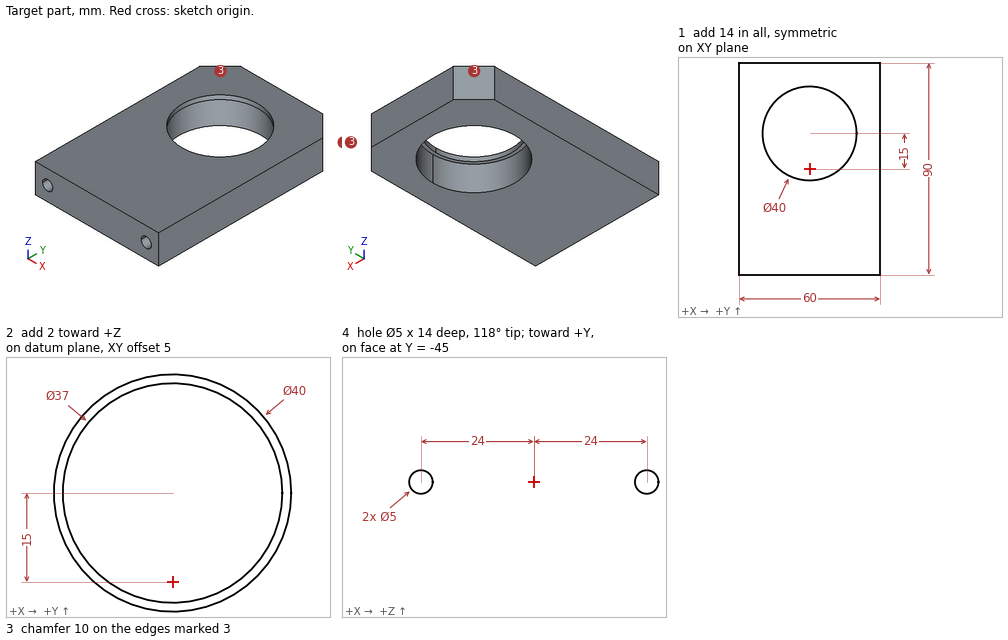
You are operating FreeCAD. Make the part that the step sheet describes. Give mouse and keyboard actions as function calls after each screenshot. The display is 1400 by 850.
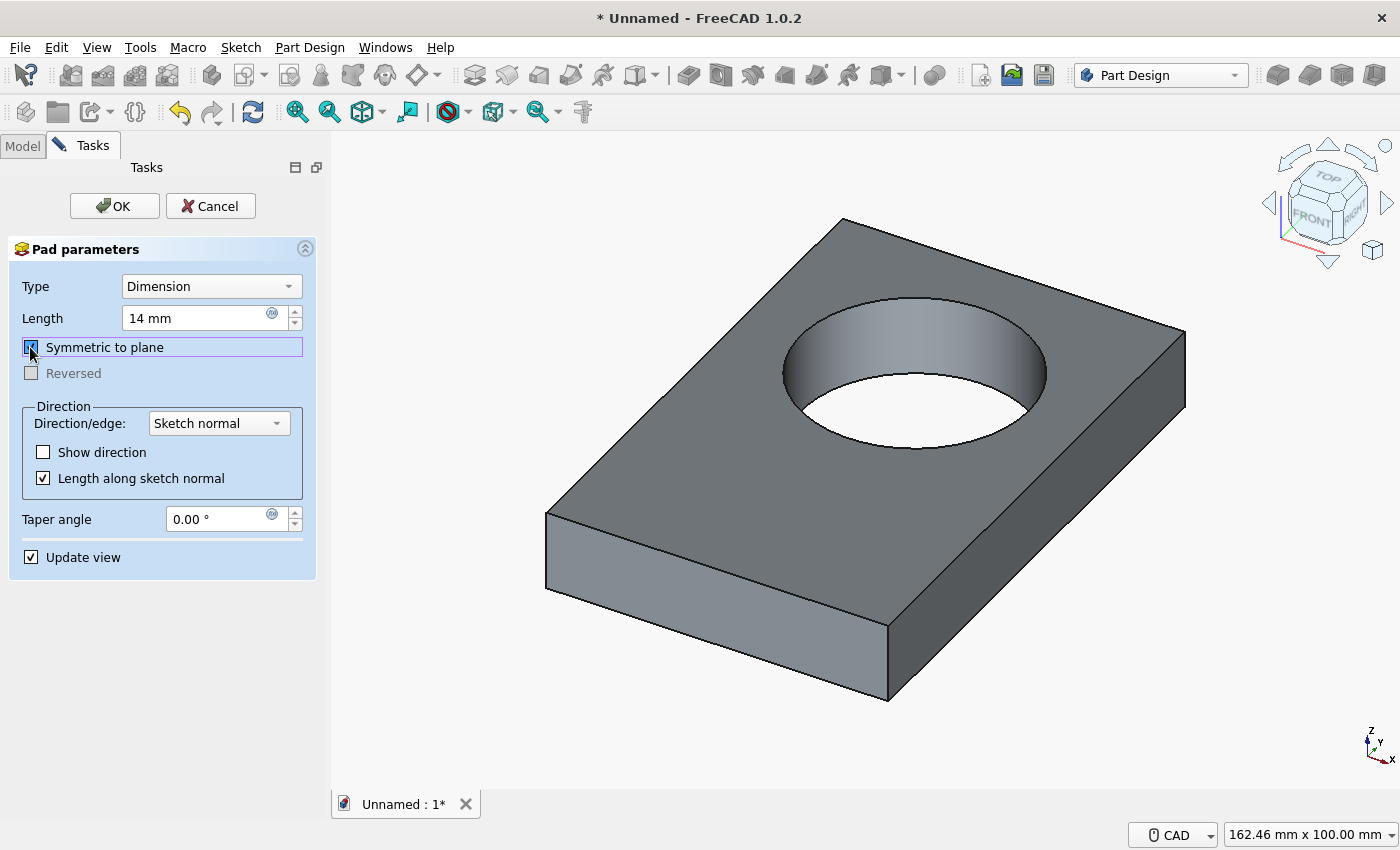
click(115, 206)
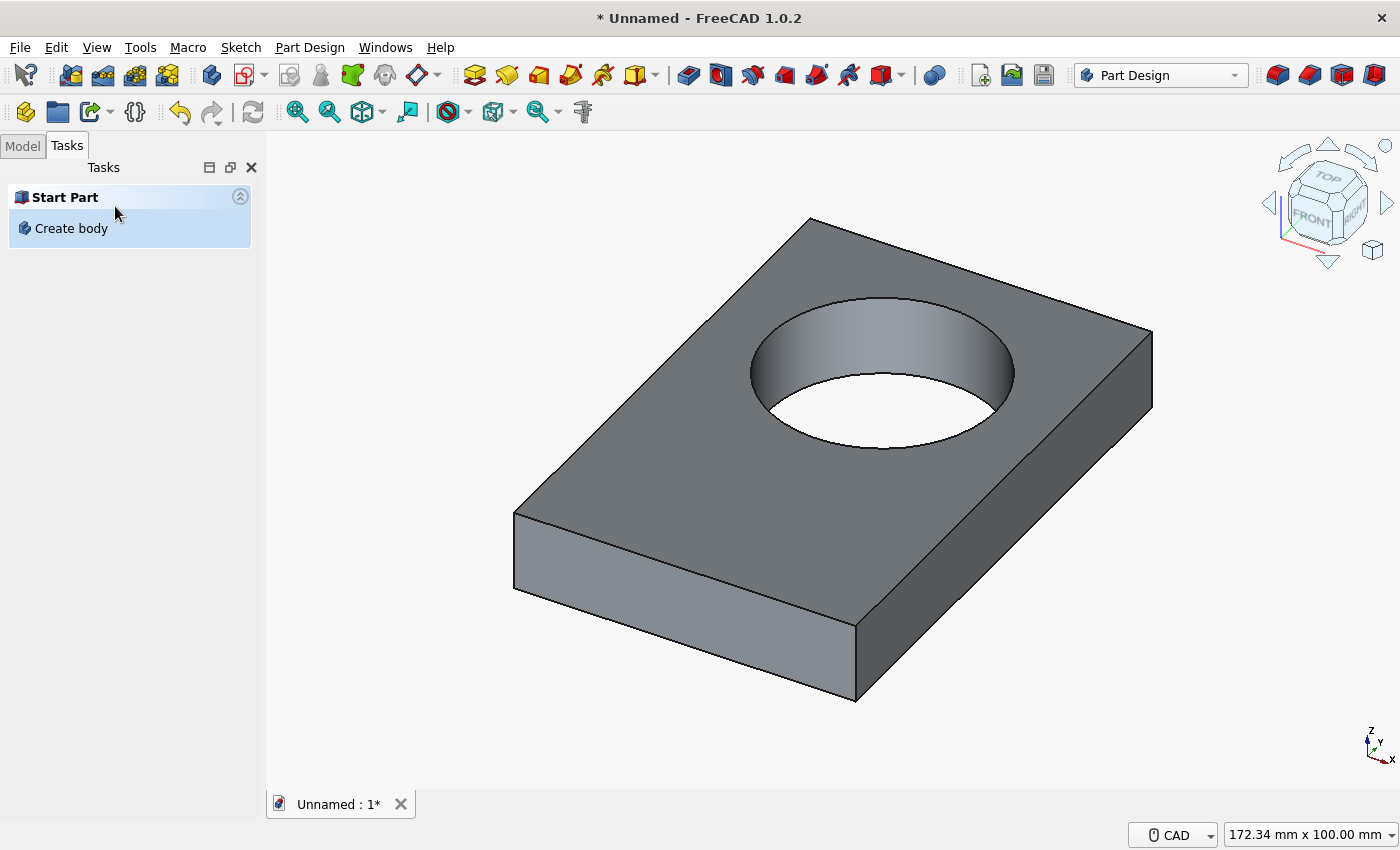
click(23, 145)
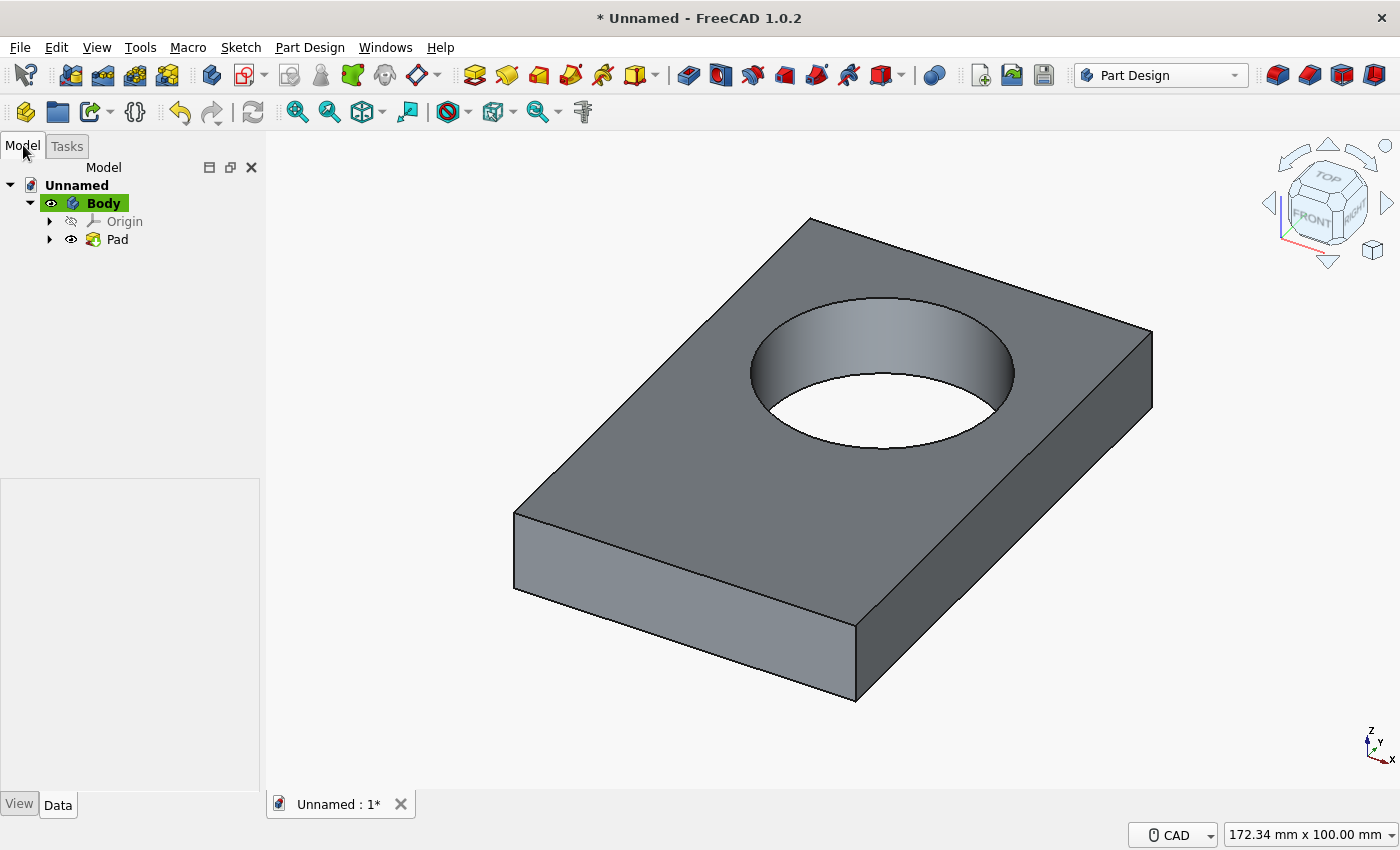
click(50, 221)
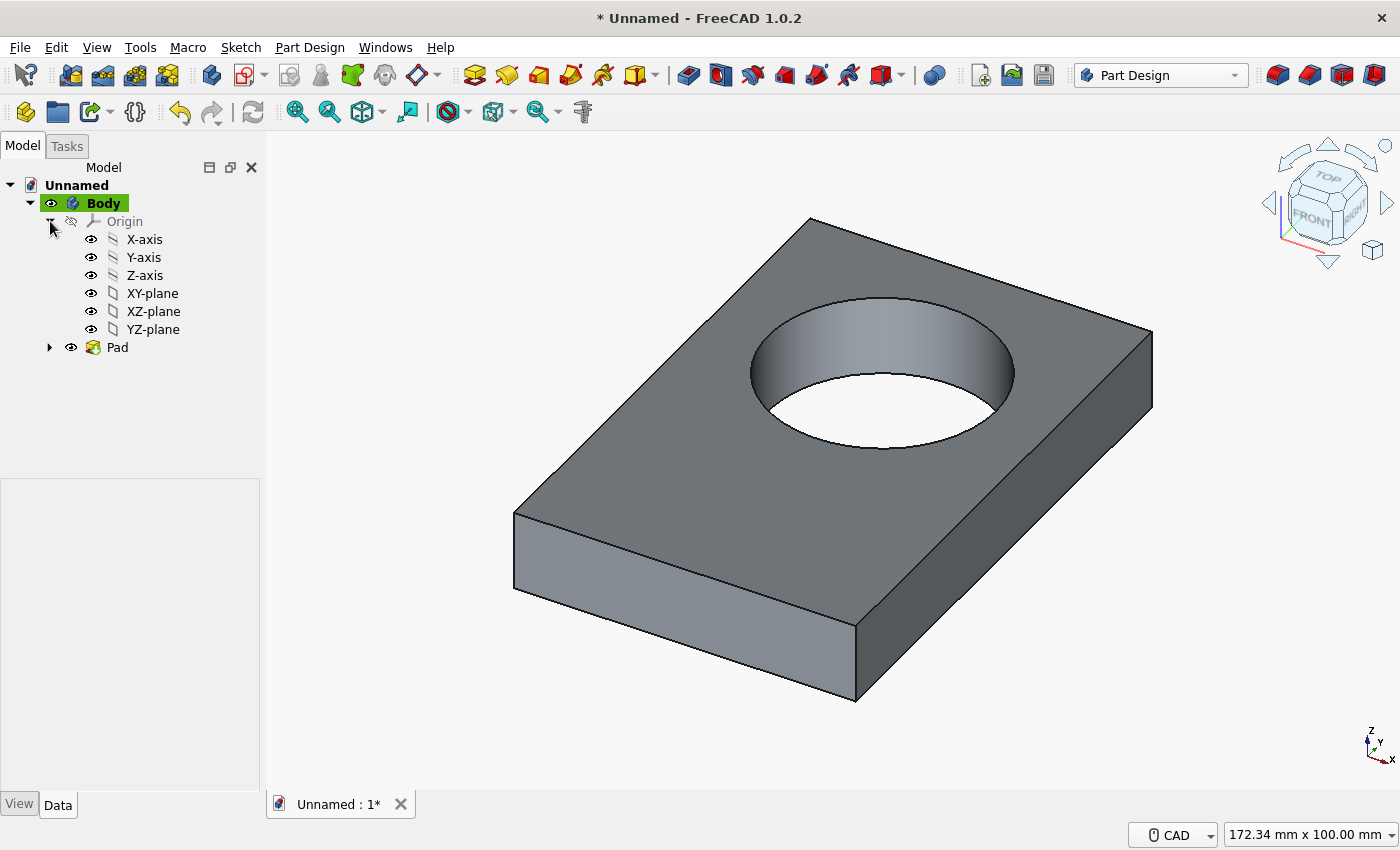
click(136, 293)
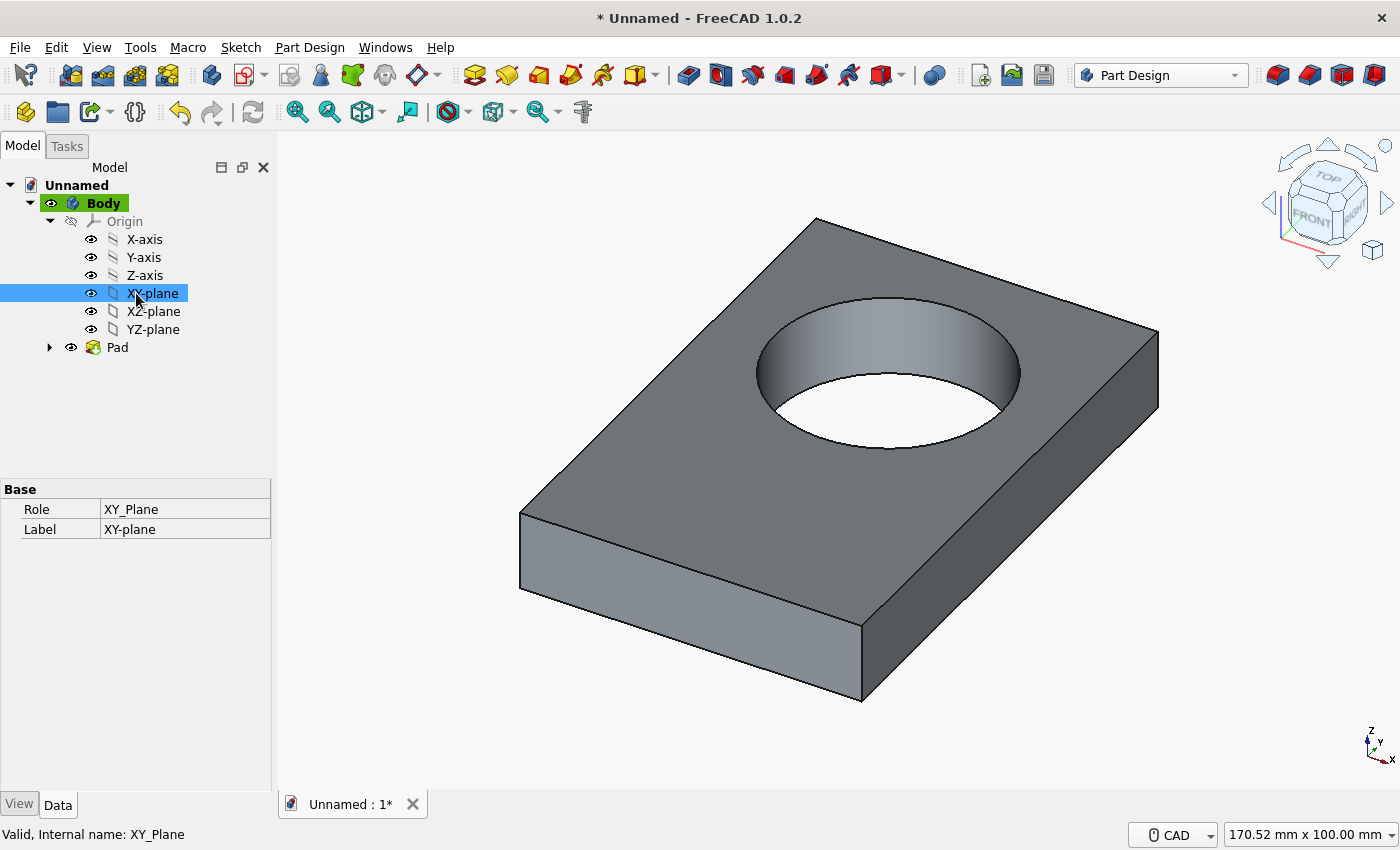
click(418, 76)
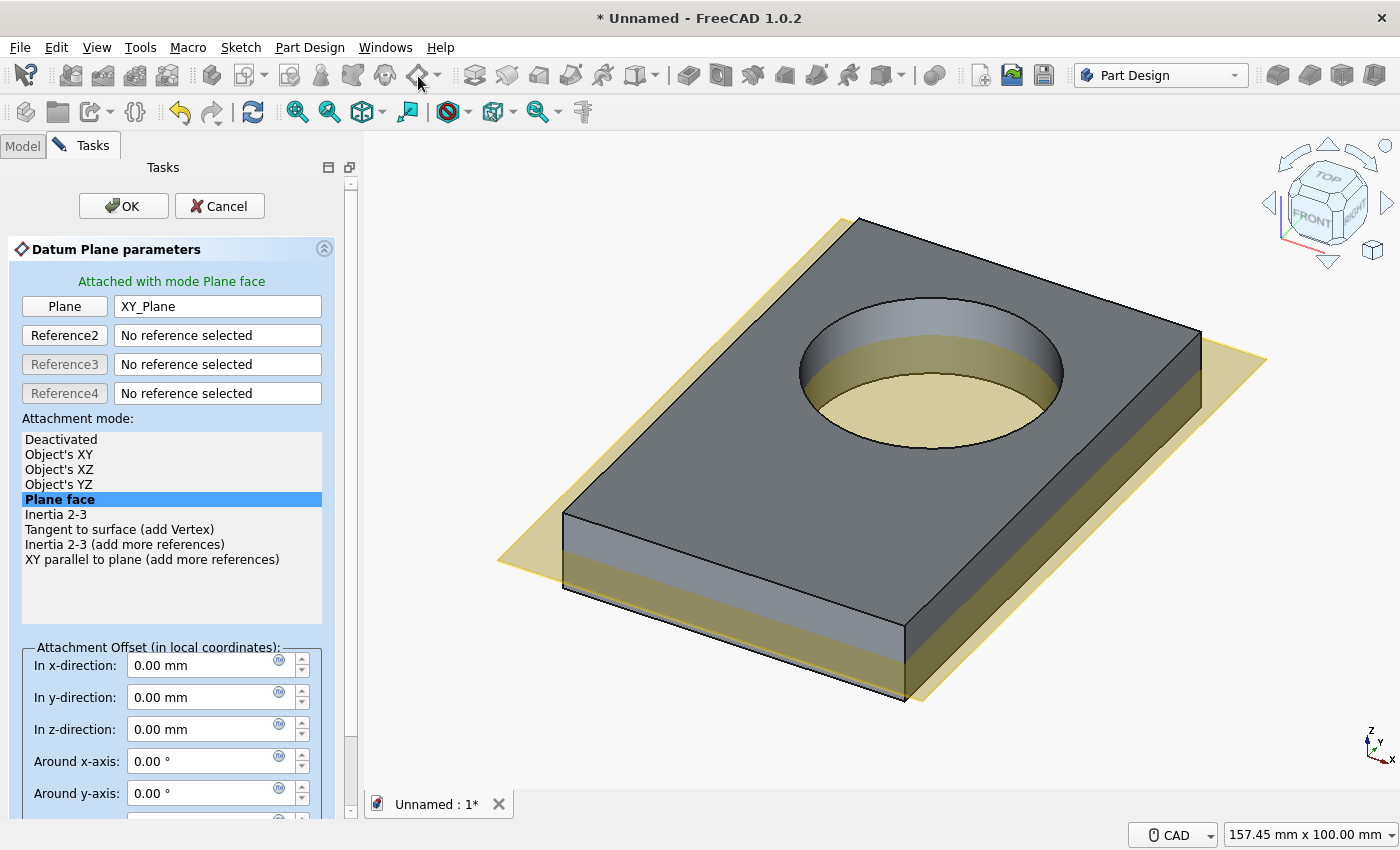
triple_click(210, 729)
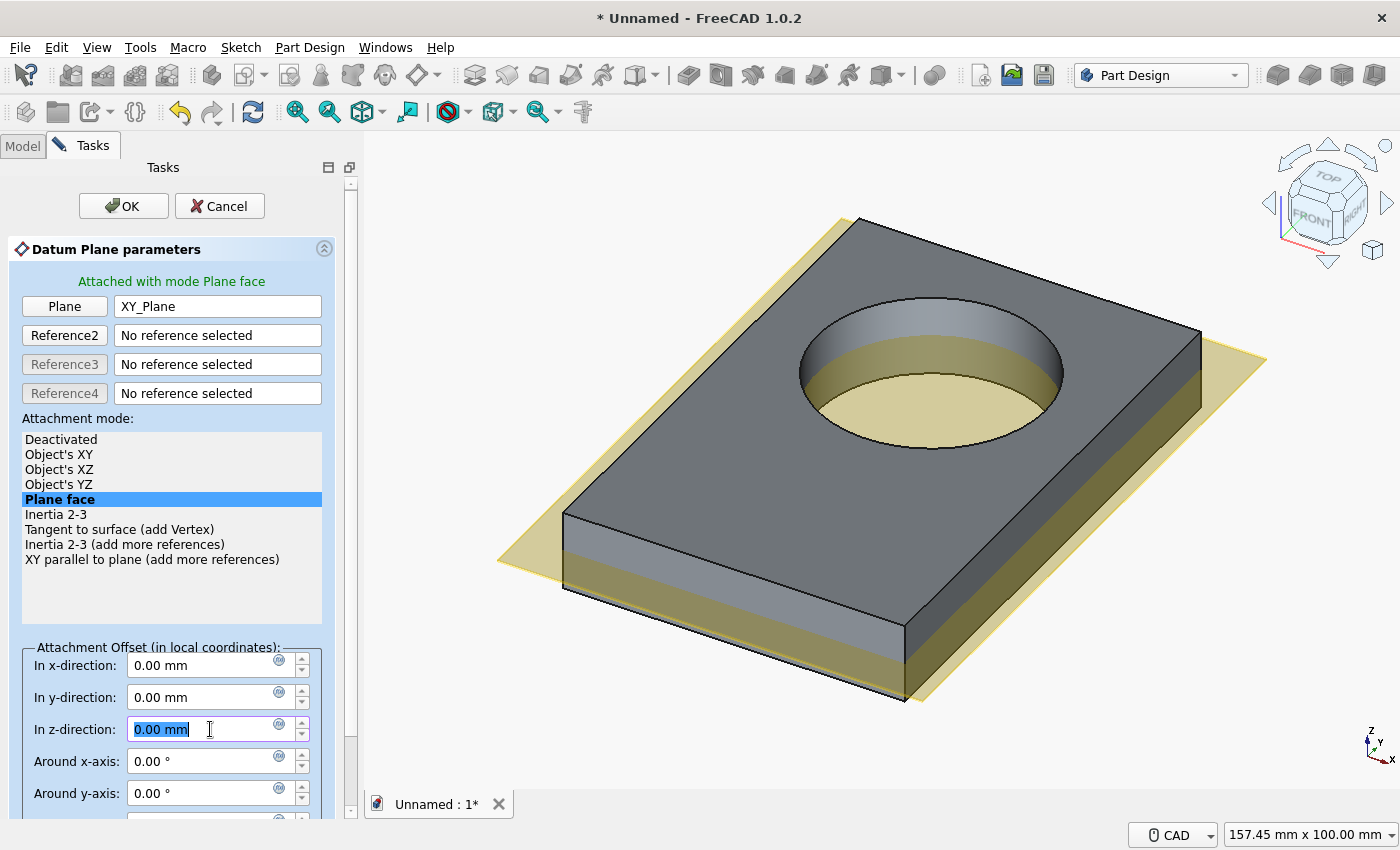
text(5)
key(Tab)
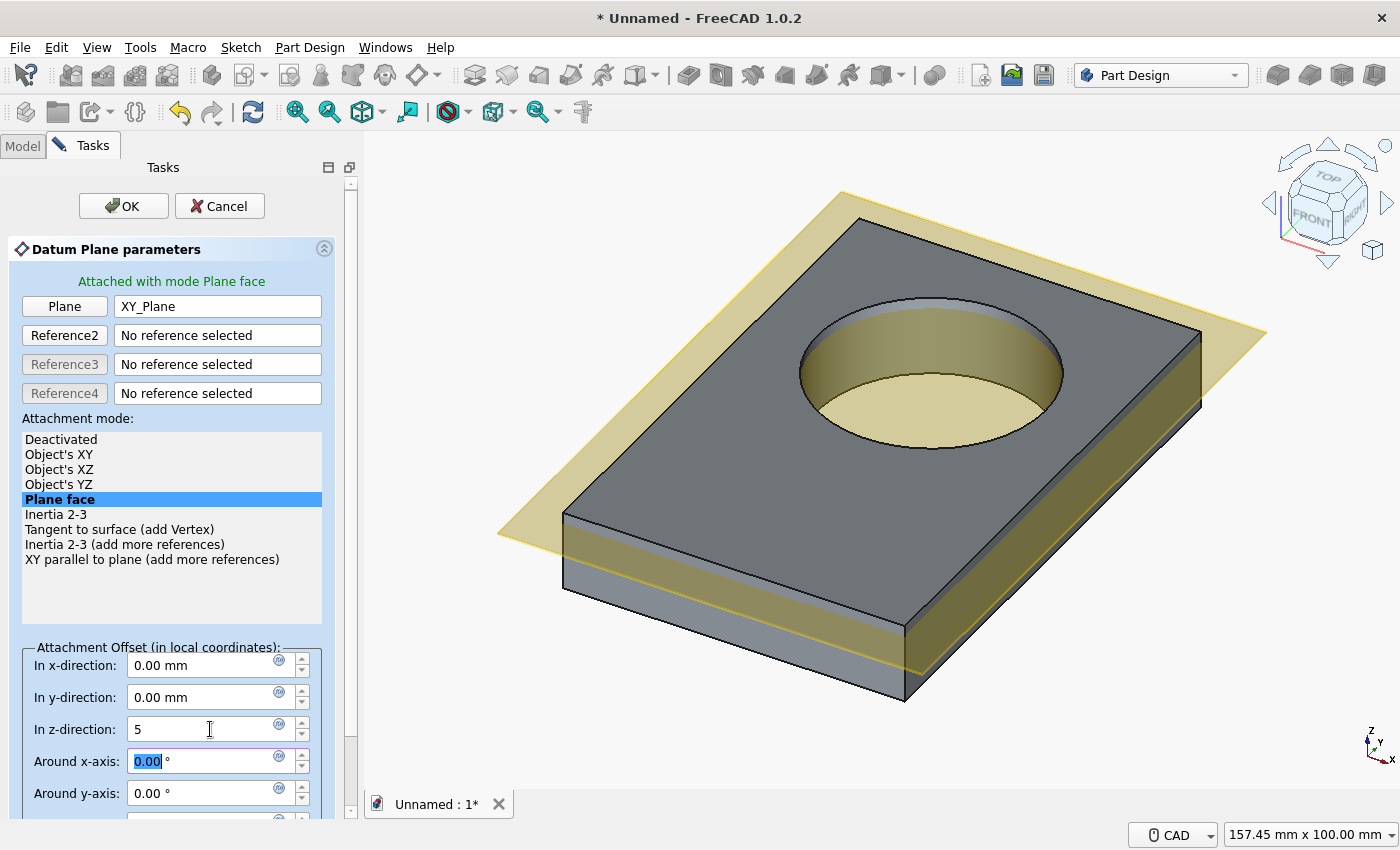
click(124, 206)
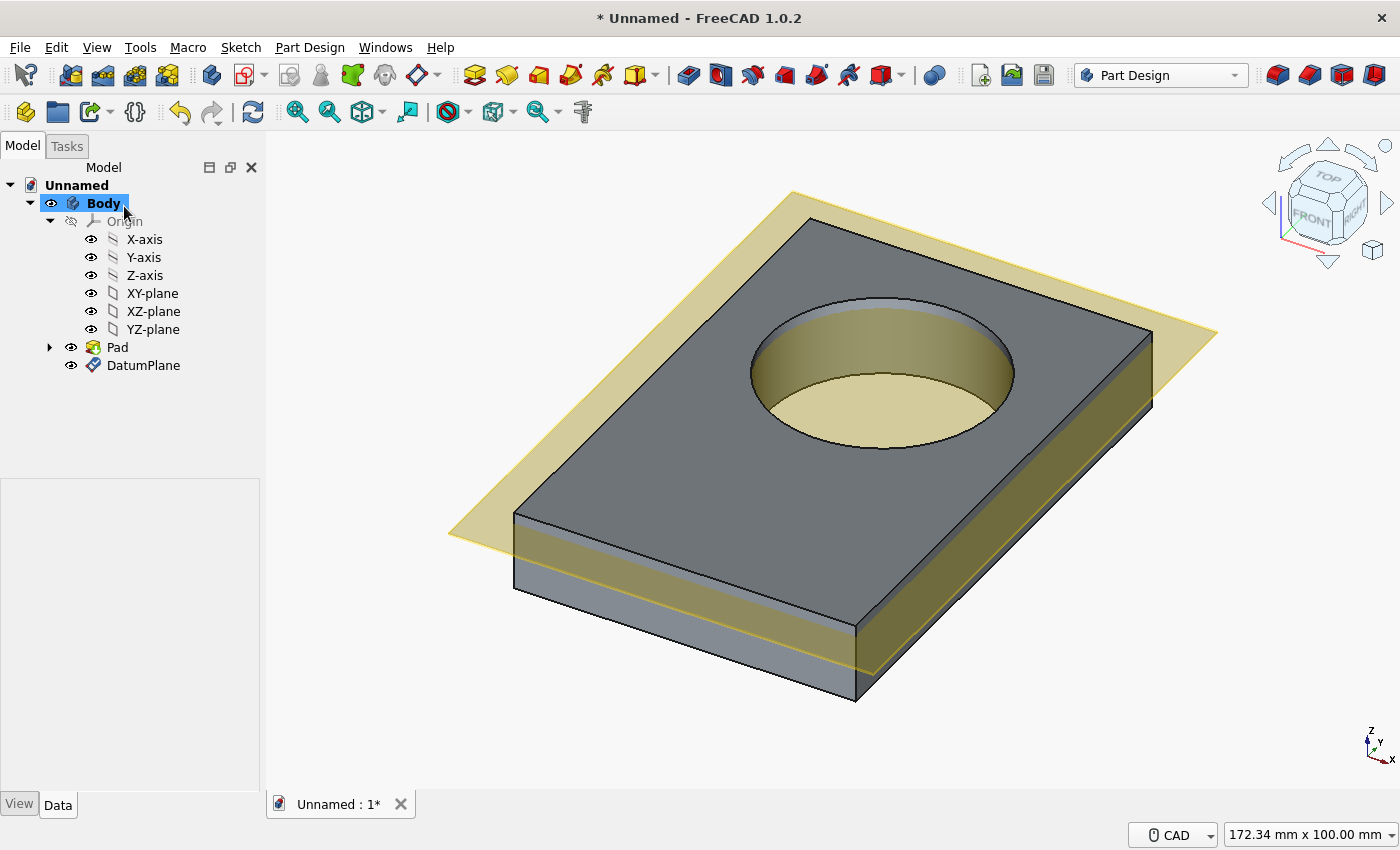
click(116, 365)